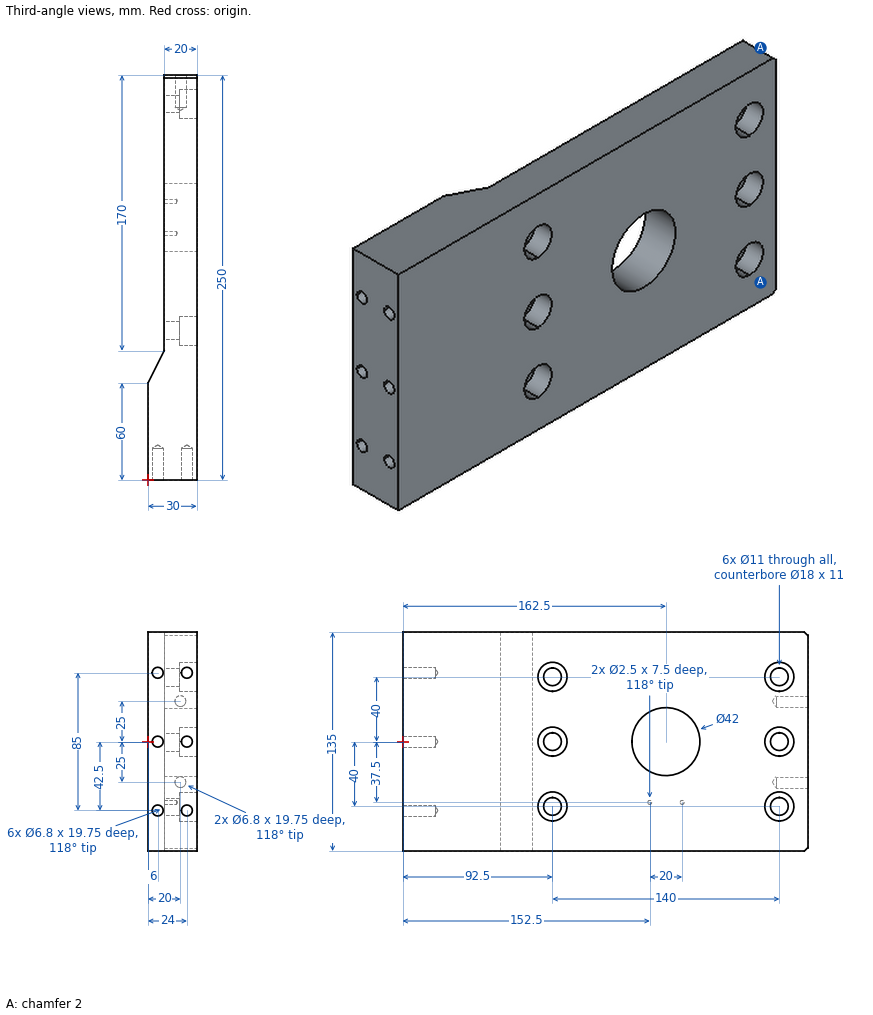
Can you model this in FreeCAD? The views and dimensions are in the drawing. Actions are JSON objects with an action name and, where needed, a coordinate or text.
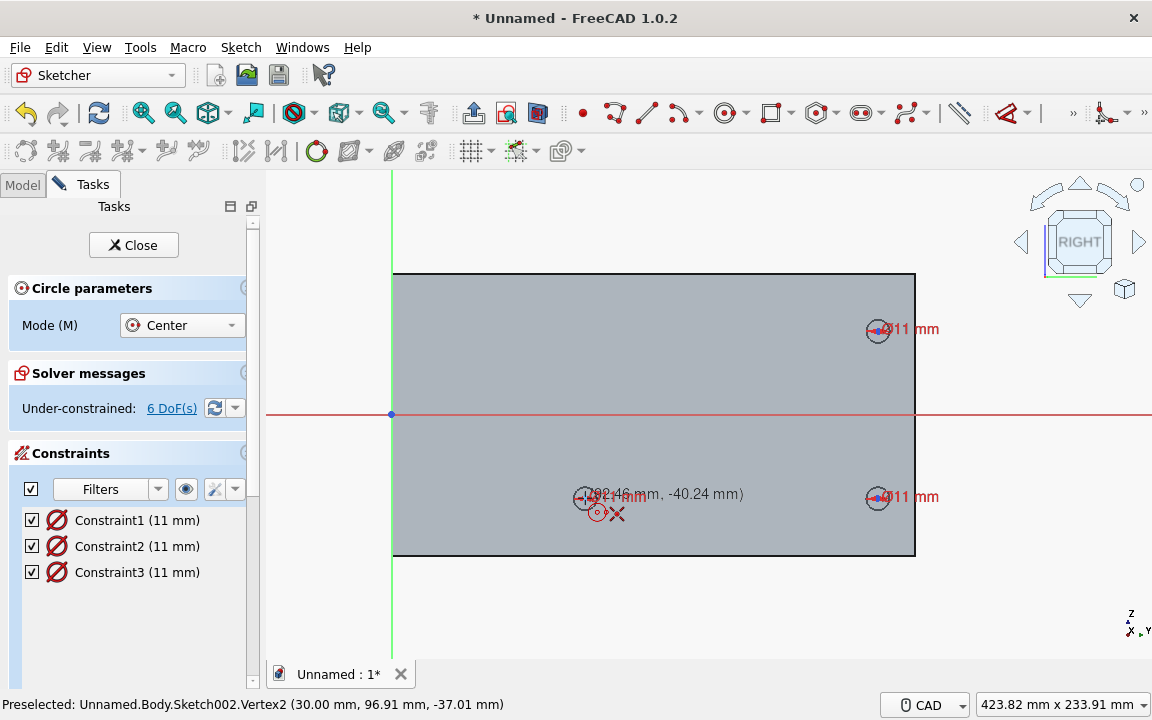
{"action": "scroll", "coordinate": [585, 331], "scroll_direction": "up", "scroll_amount": 4}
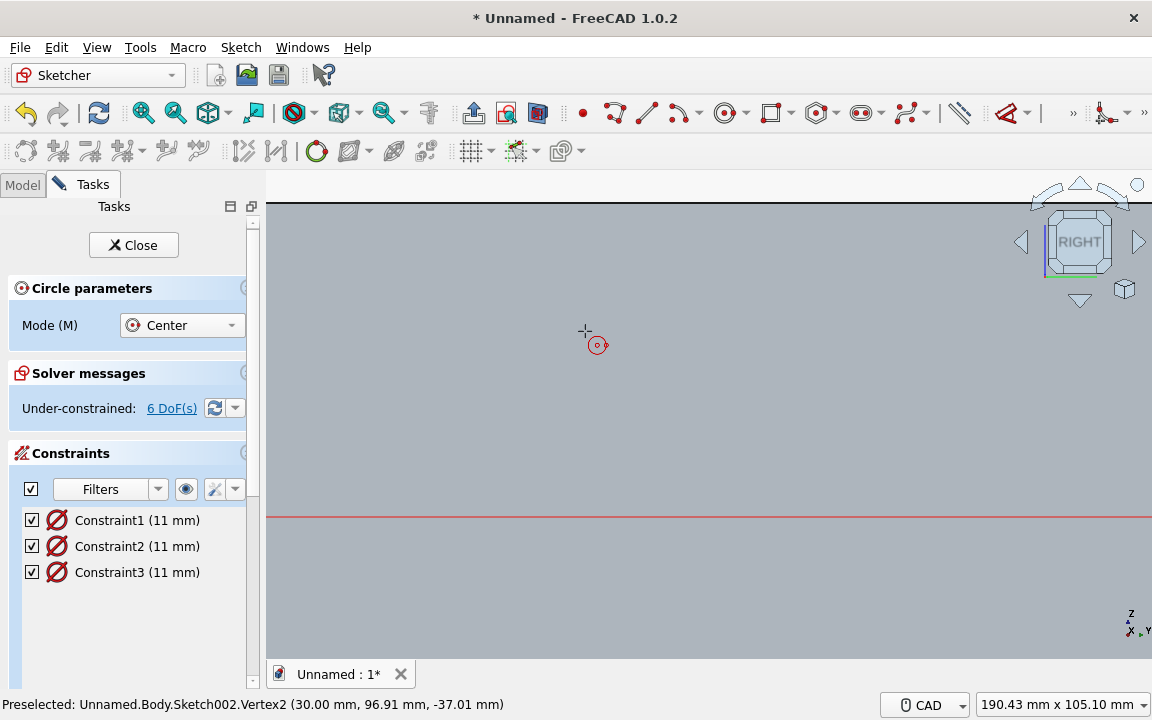
{"action": "left_click", "coordinate": [585, 331]}
{"action": "mouse_move", "coordinate": [603, 313]}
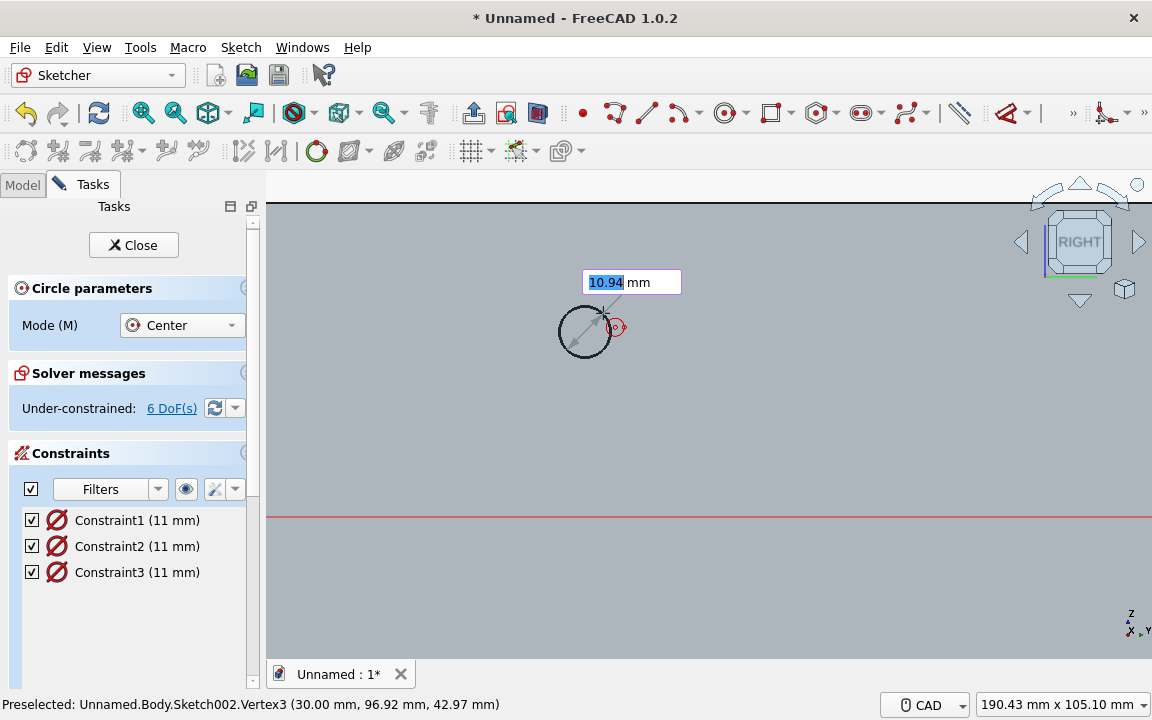
{"action": "type", "text": "11"}
{"action": "key", "text": "Return"}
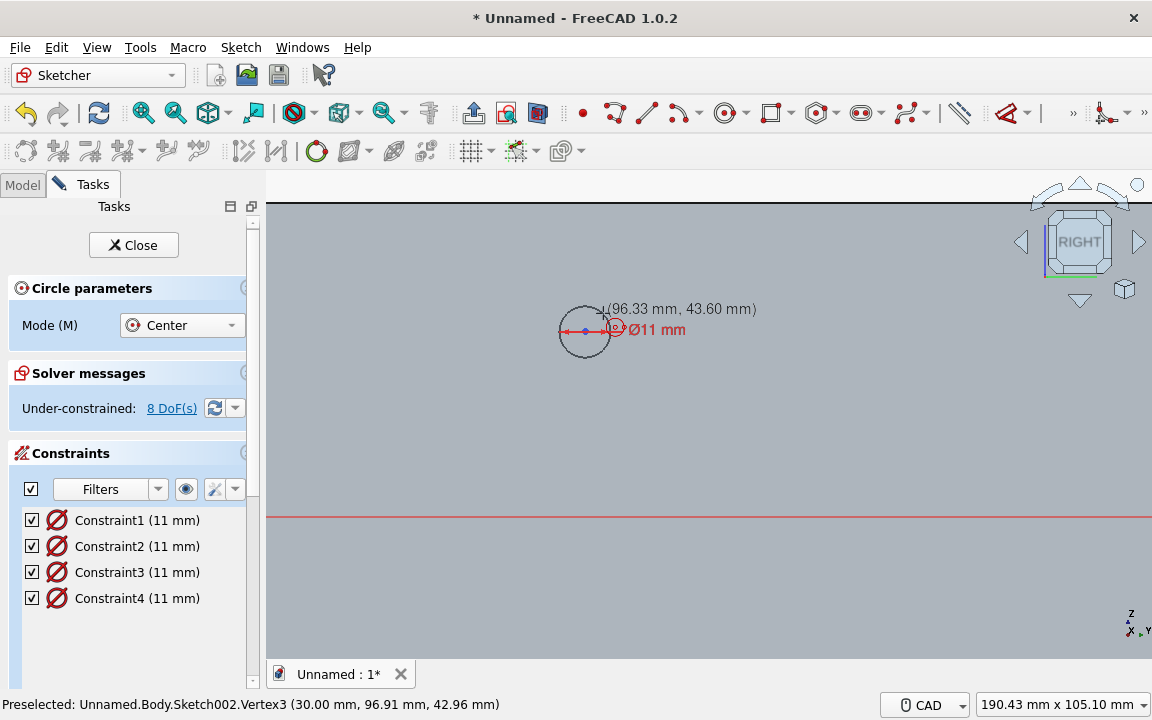
{"action": "scroll", "coordinate": [585, 331], "scroll_direction": "down", "scroll_amount": 4}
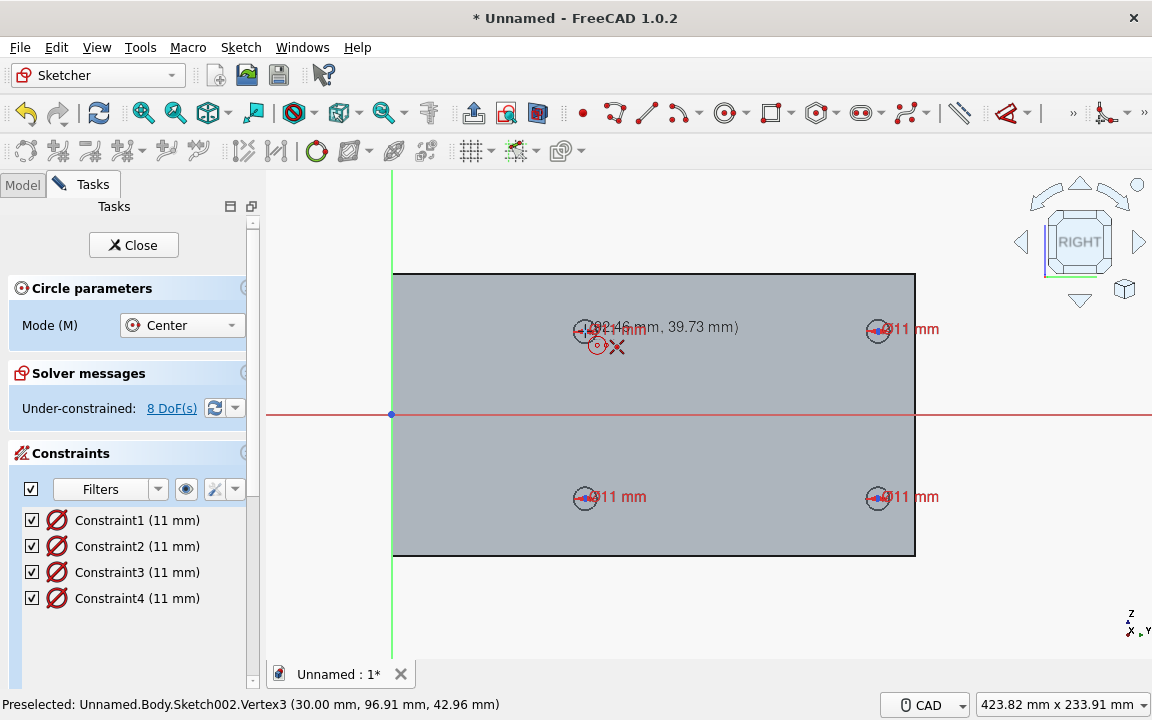
{"action": "scroll", "coordinate": [878, 415], "scroll_direction": "up", "scroll_amount": 4}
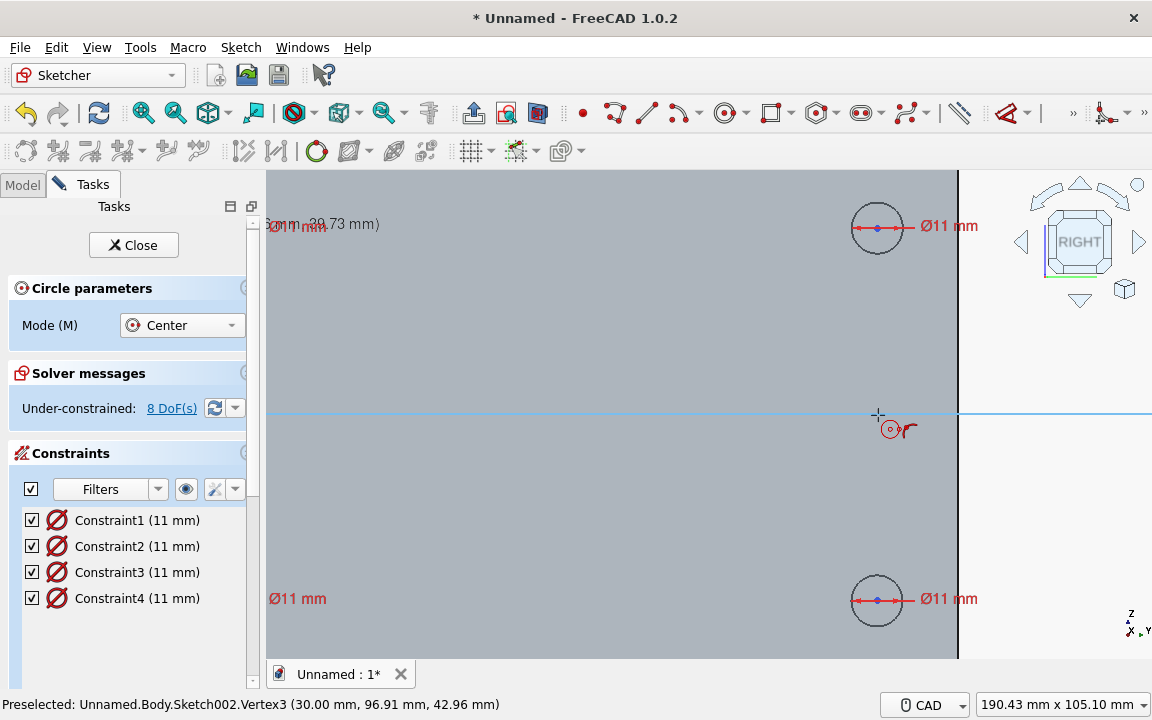
{"action": "left_click", "coordinate": [877, 414]}
{"action": "mouse_move", "coordinate": [895, 396]}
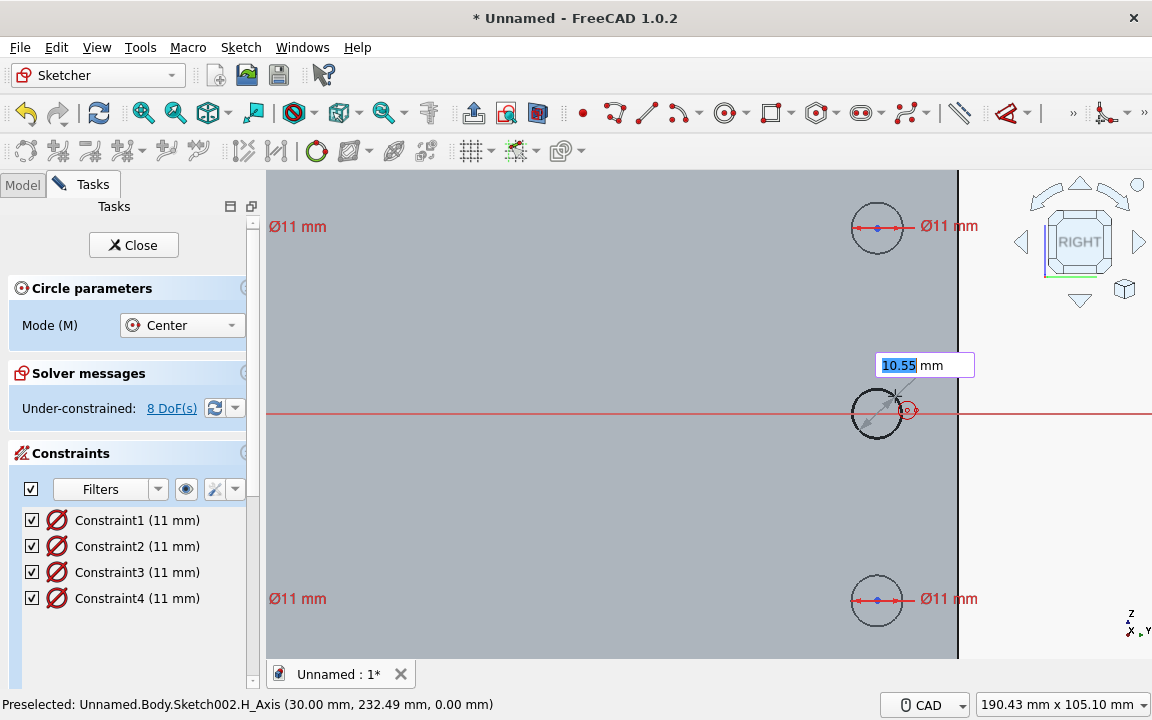
{"action": "type", "text": "11"}
{"action": "key", "text": "Return"}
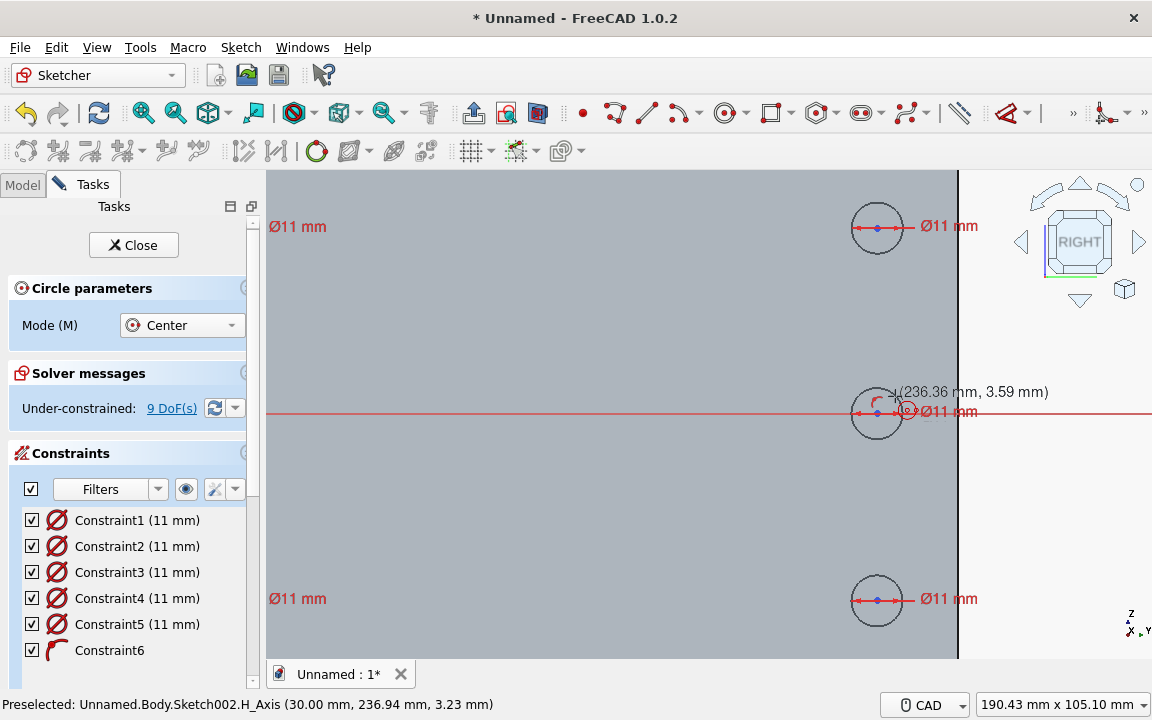
{"action": "scroll", "coordinate": [878, 415], "scroll_direction": "down", "scroll_amount": 4}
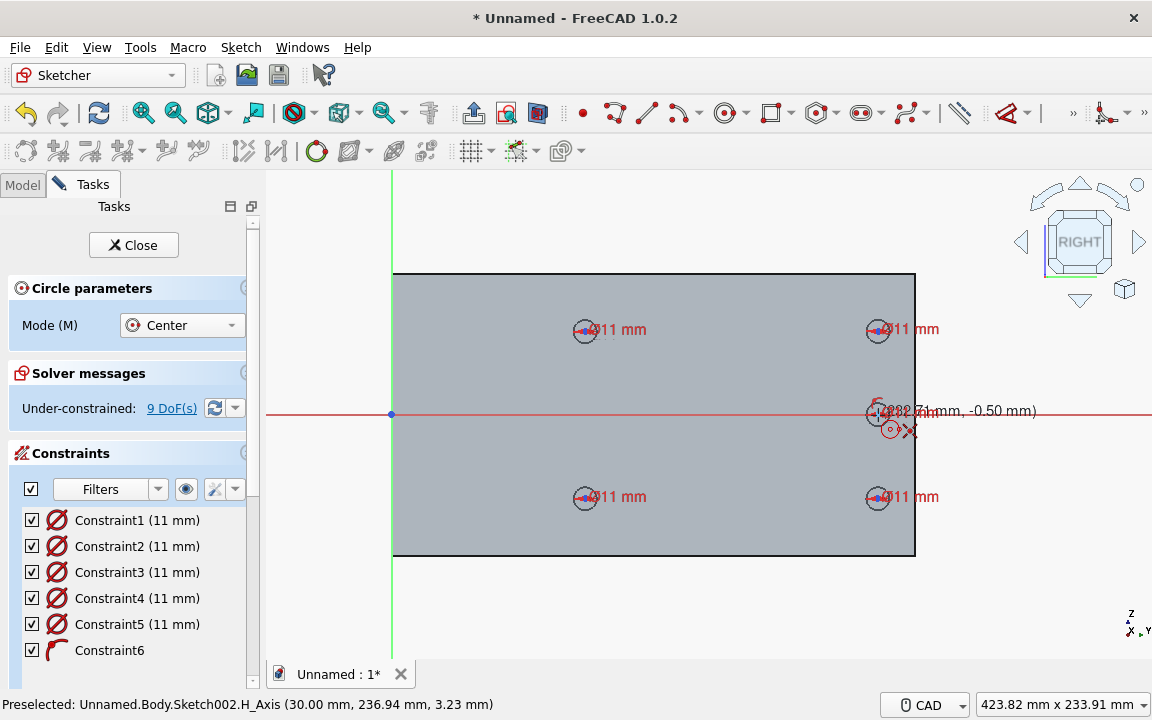
{"action": "scroll", "coordinate": [585, 415], "scroll_direction": "up", "scroll_amount": 4}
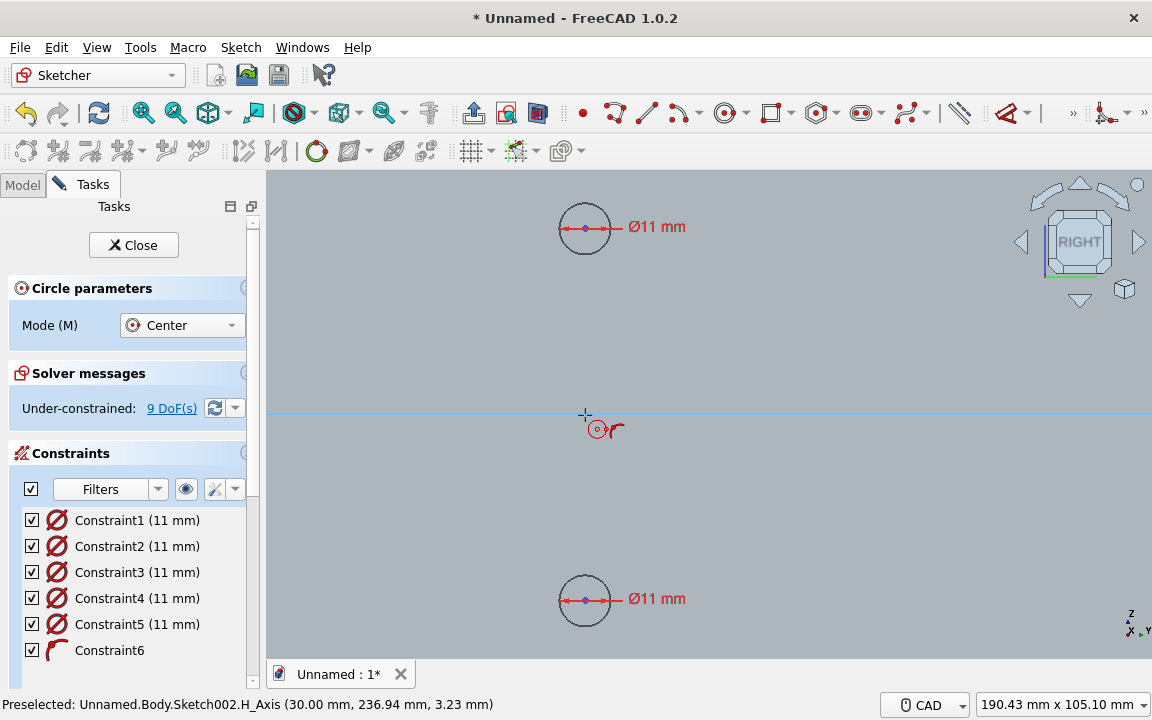
{"action": "left_click", "coordinate": [585, 414]}
{"action": "mouse_move", "coordinate": [603, 396]}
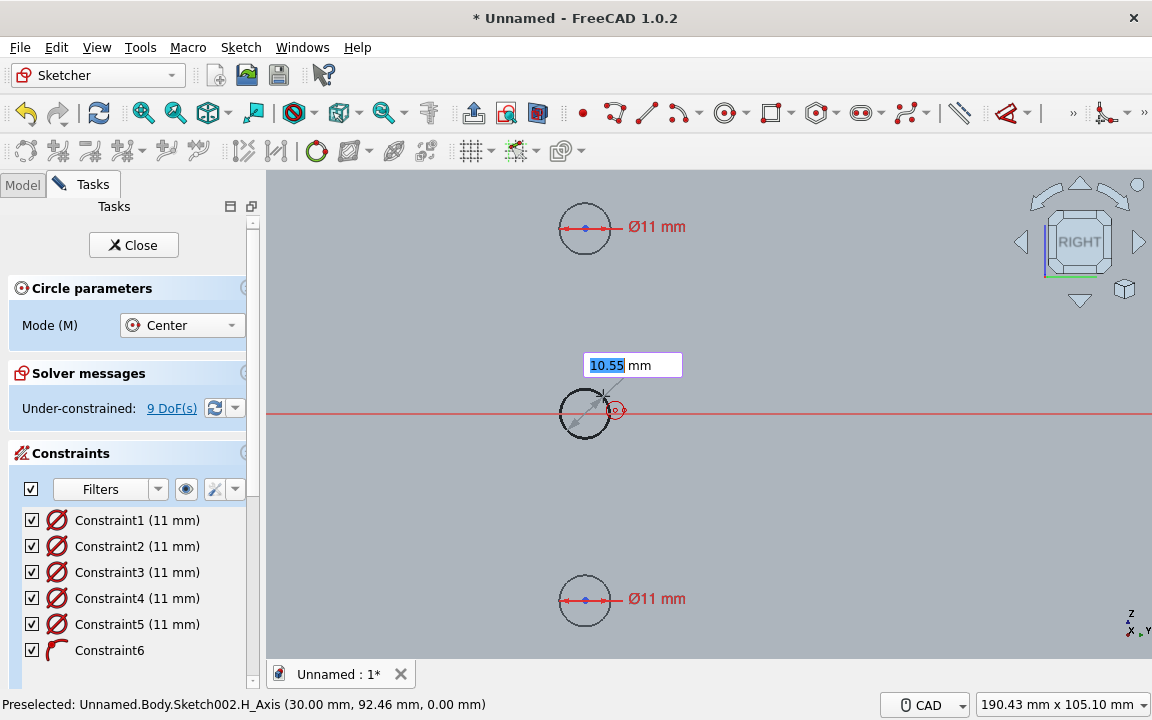
{"action": "type", "text": "11"}
{"action": "key", "text": "Return"}
{"action": "key", "text": "Escape"}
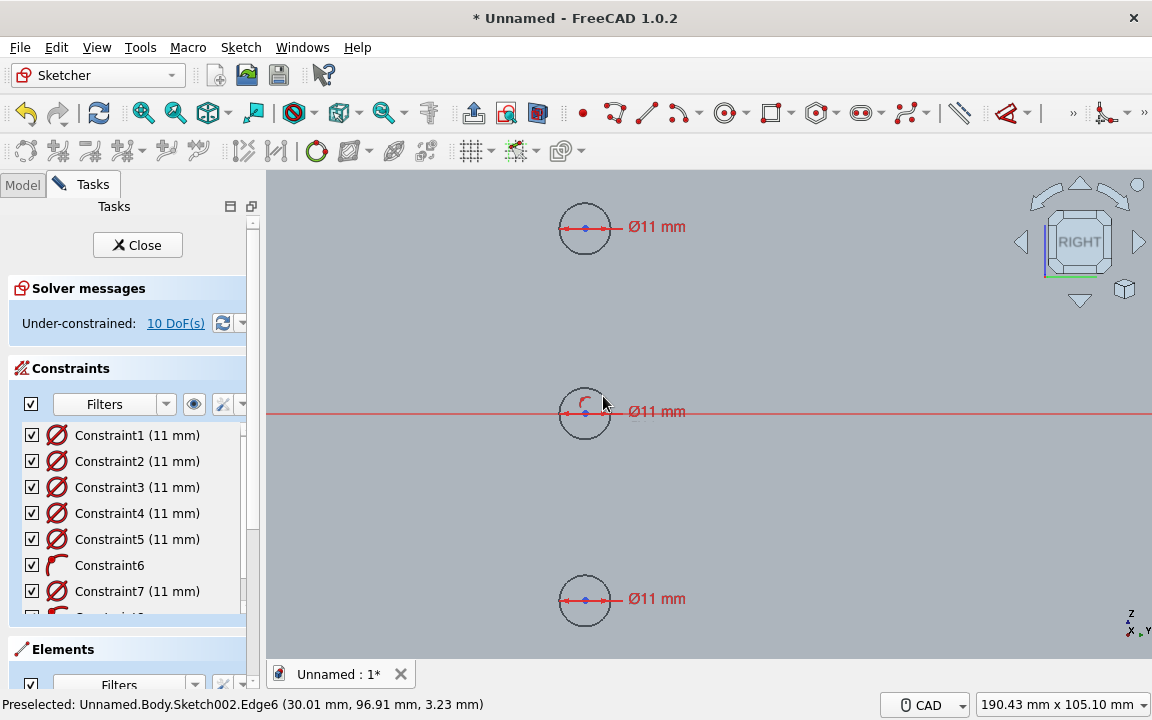
{"action": "scroll", "coordinate": [585, 415], "scroll_direction": "down", "scroll_amount": 4}